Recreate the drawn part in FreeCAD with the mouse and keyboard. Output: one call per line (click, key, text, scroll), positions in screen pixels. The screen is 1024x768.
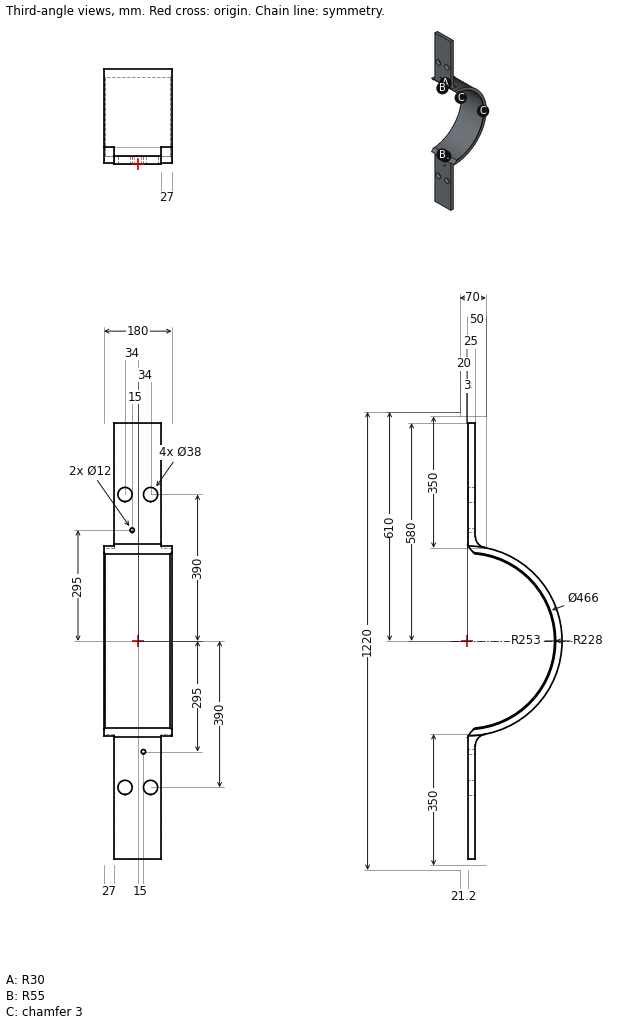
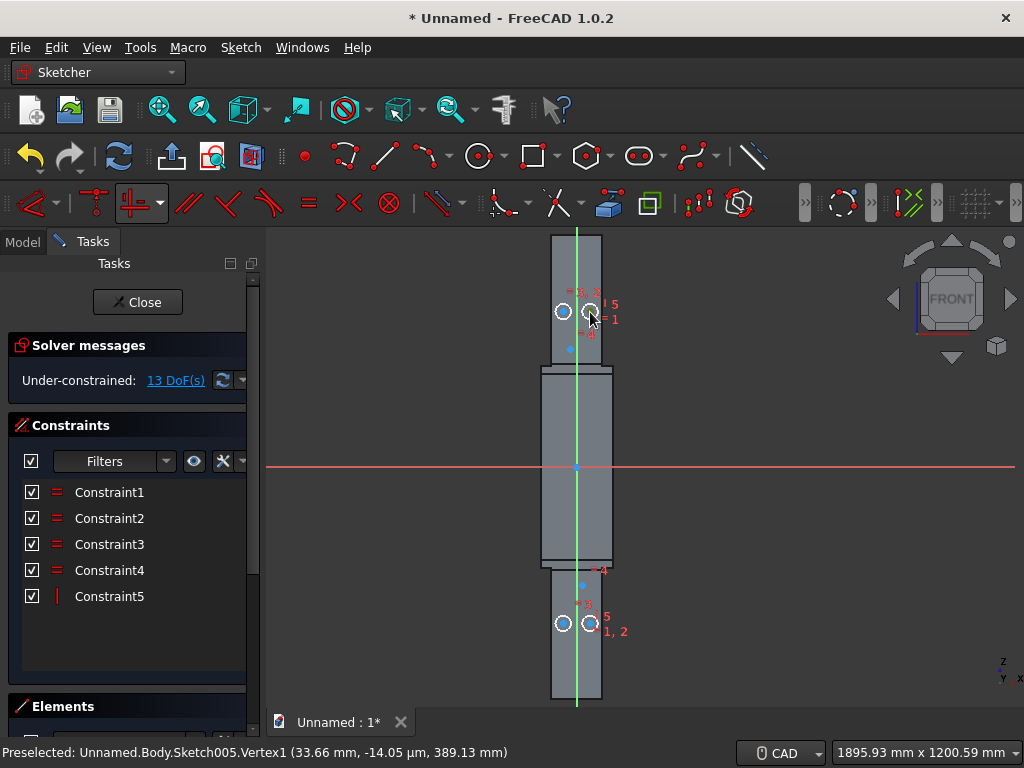
click(563, 312)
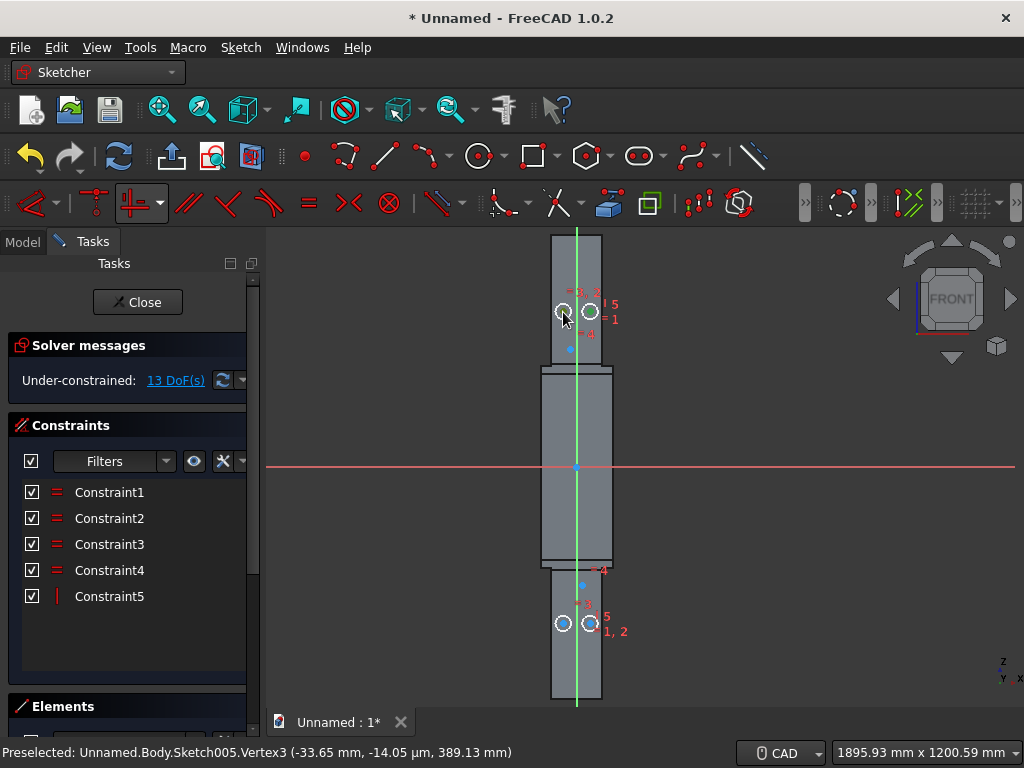
key(h)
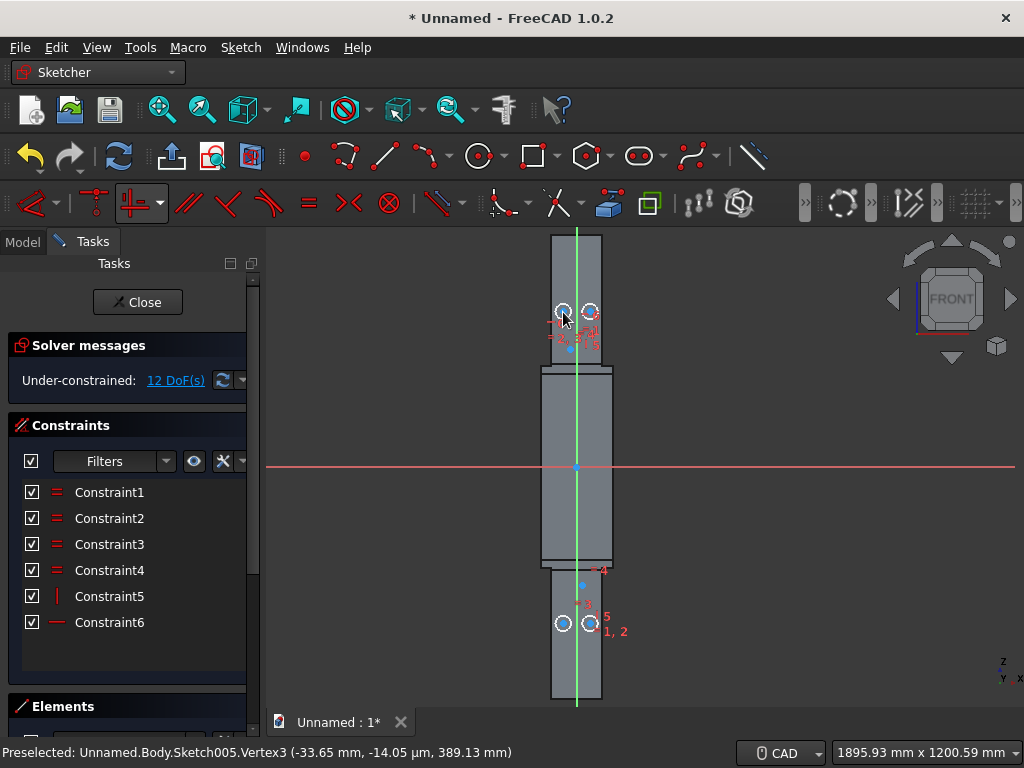
click(563, 312)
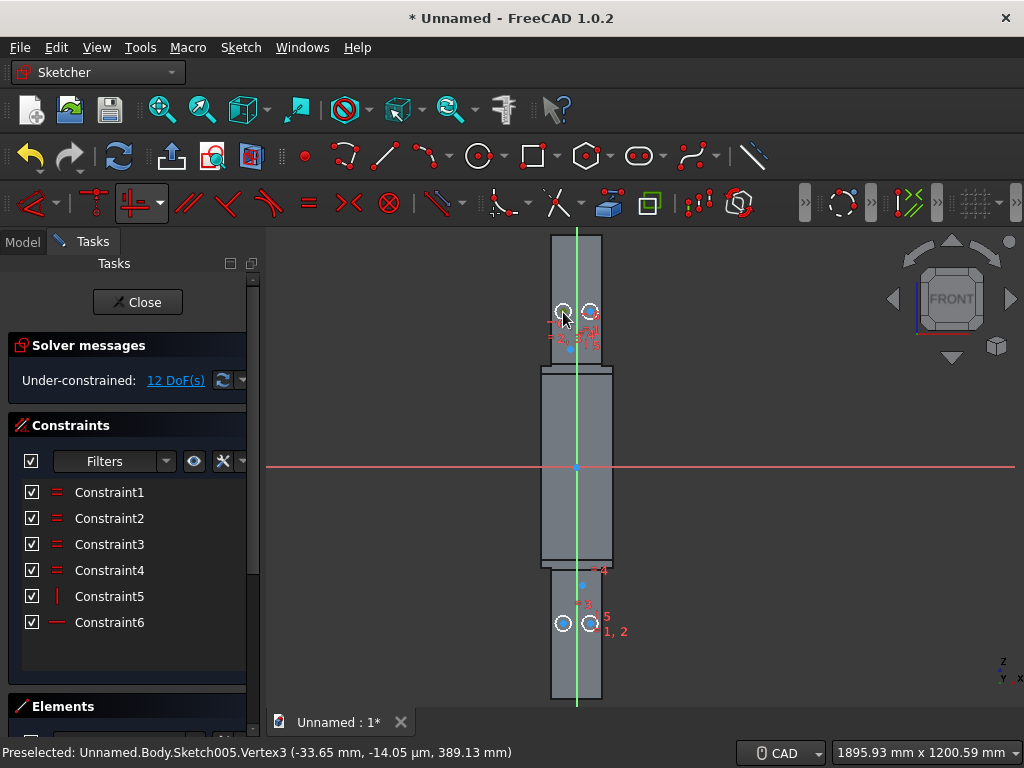
click(563, 623)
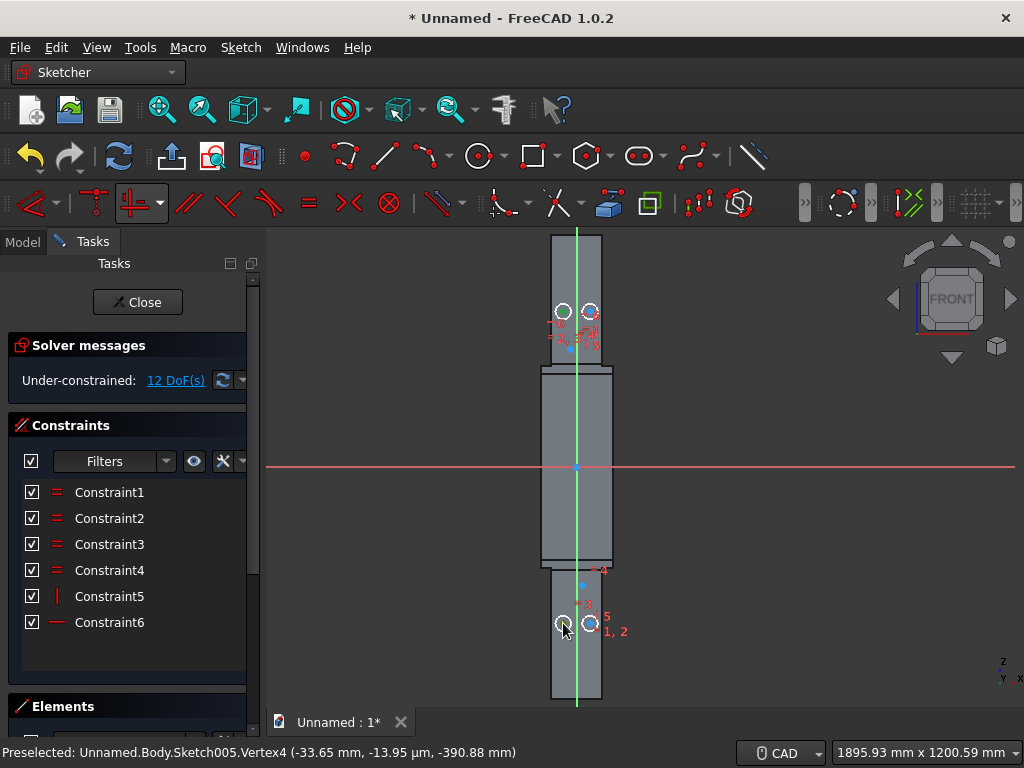
key(v)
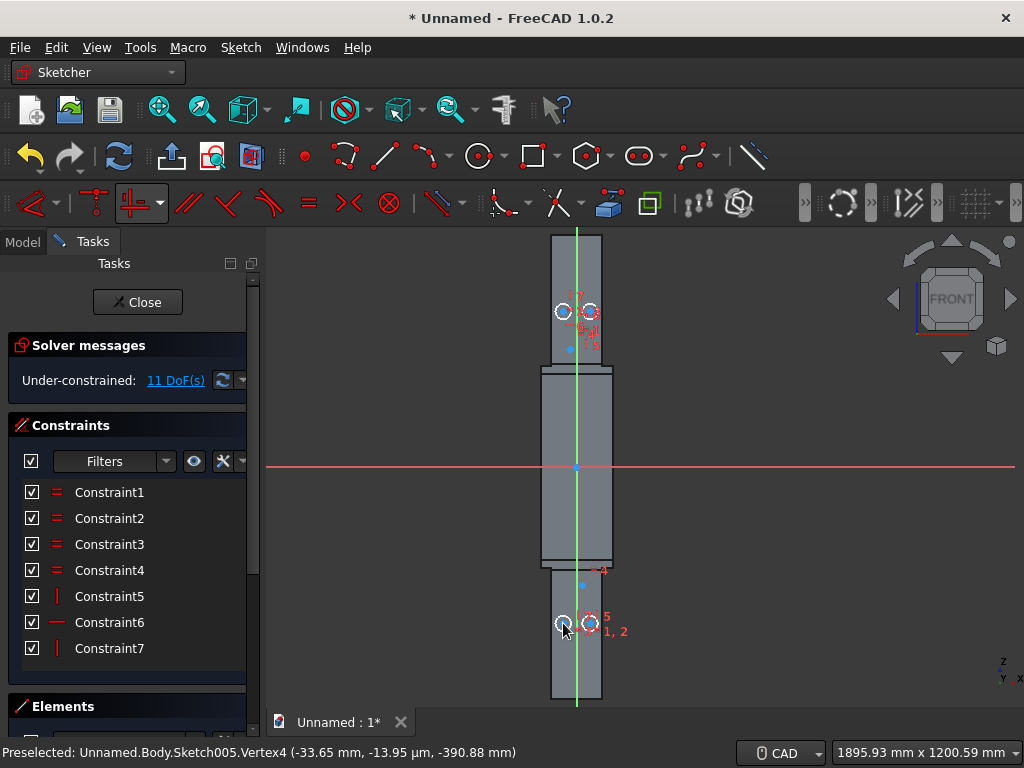
scroll(590, 623, up, 4)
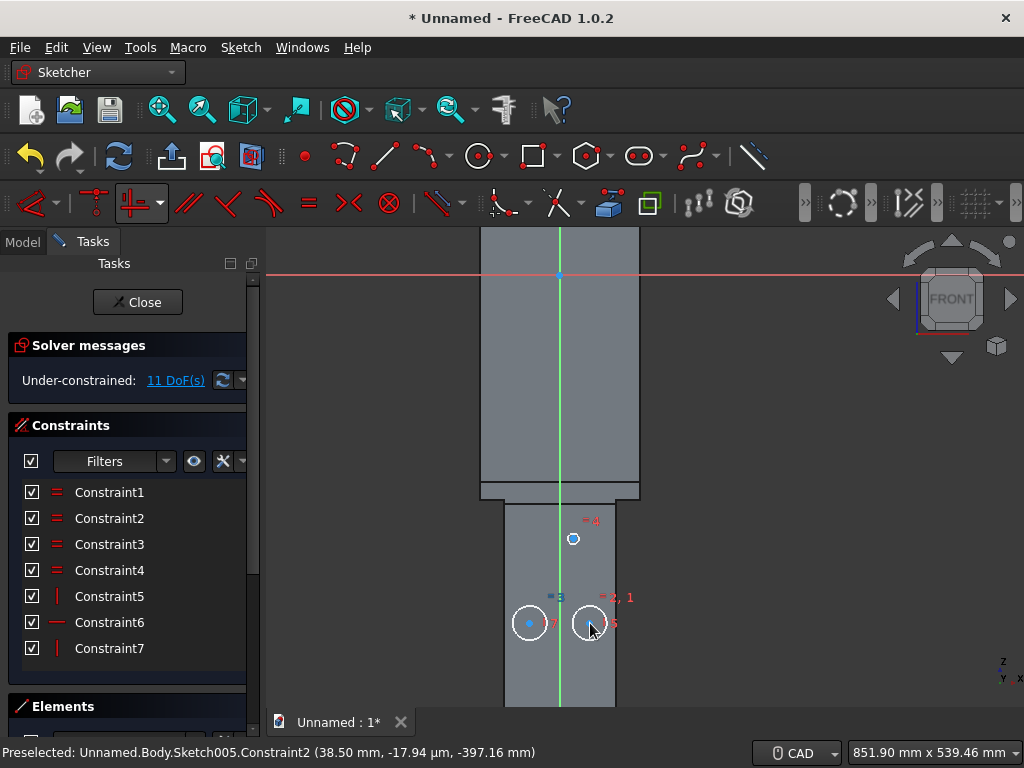
click(590, 623)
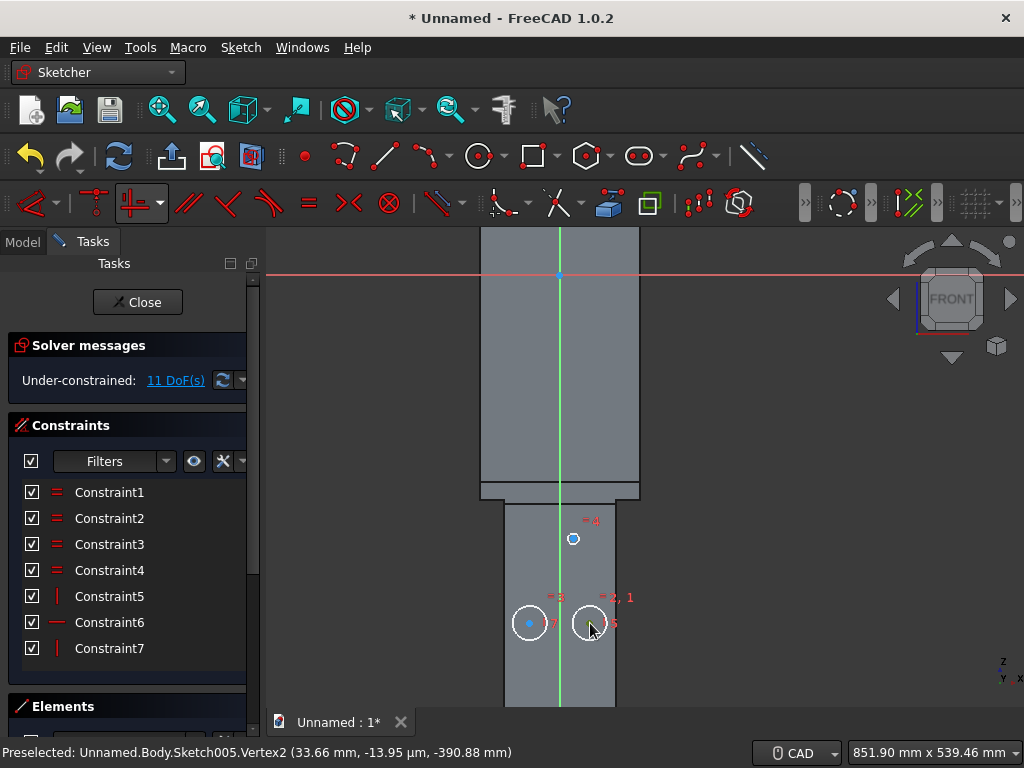
click(530, 623)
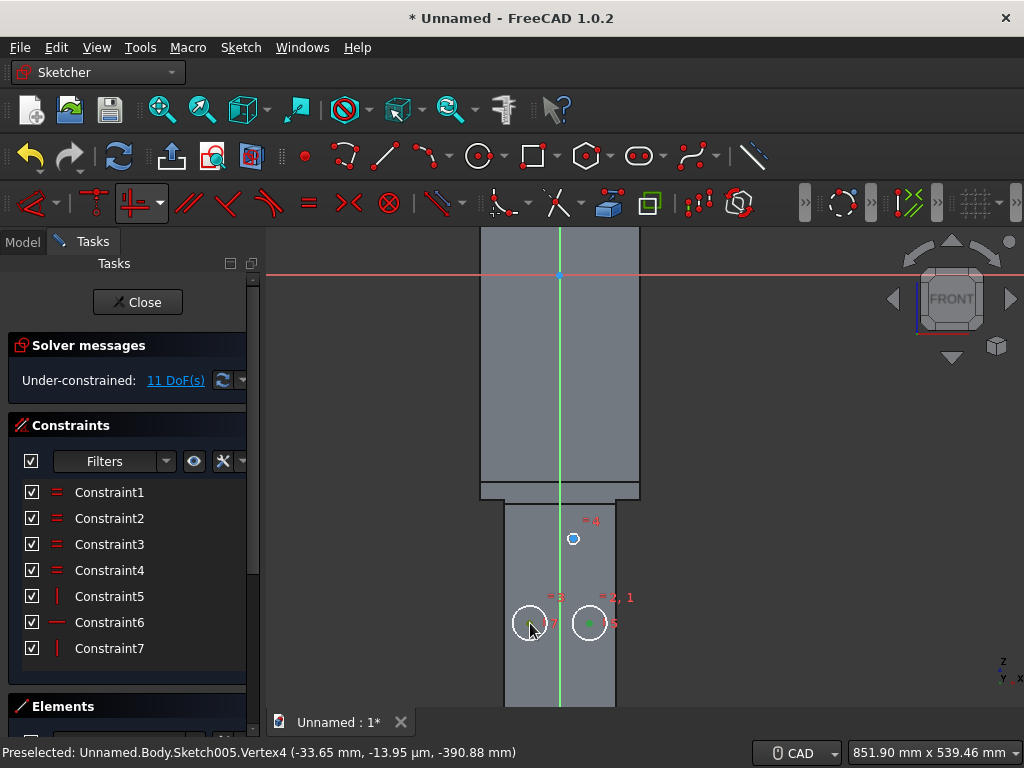
key(h)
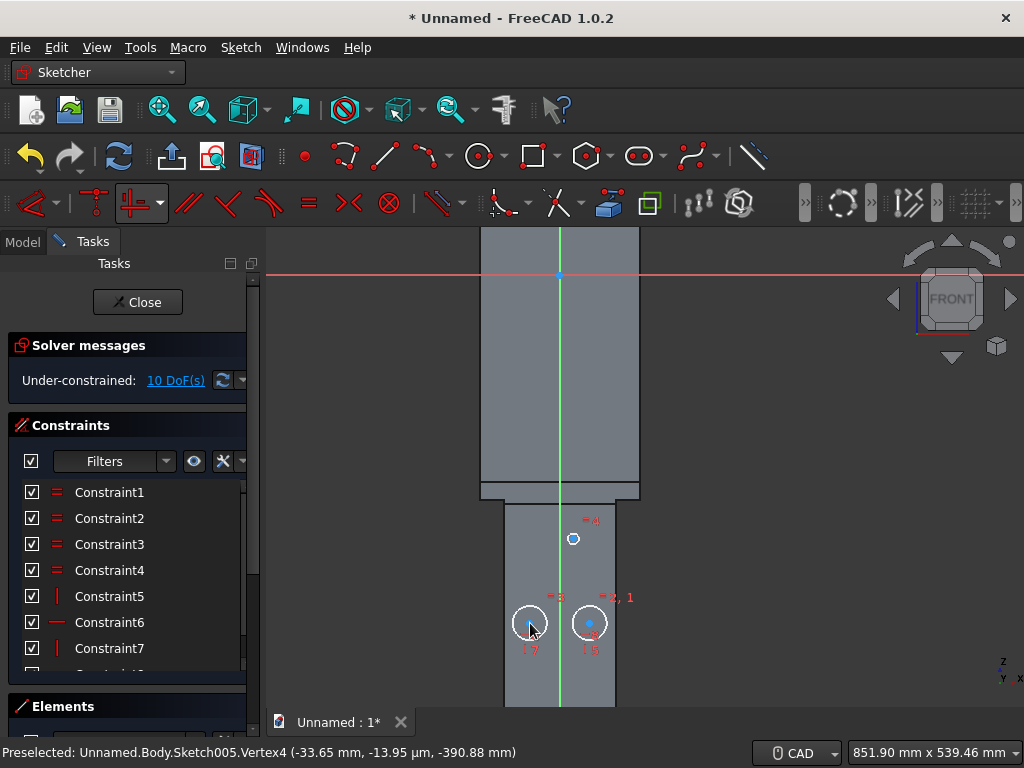
click(32, 204)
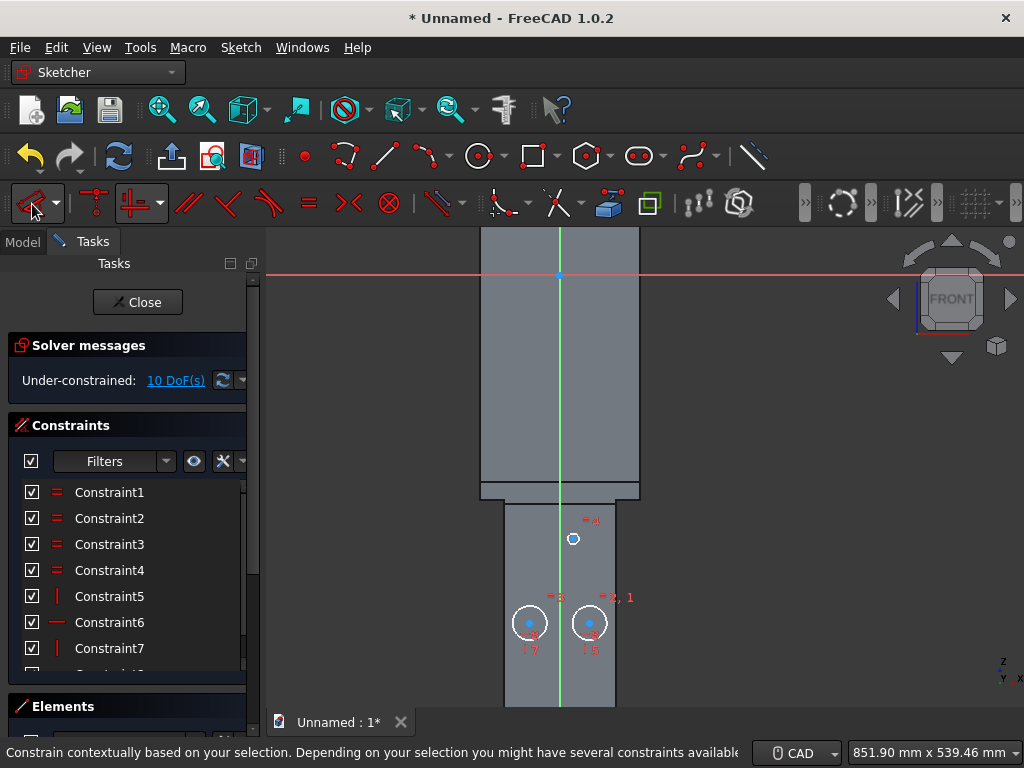
scroll(590, 623, down, 4)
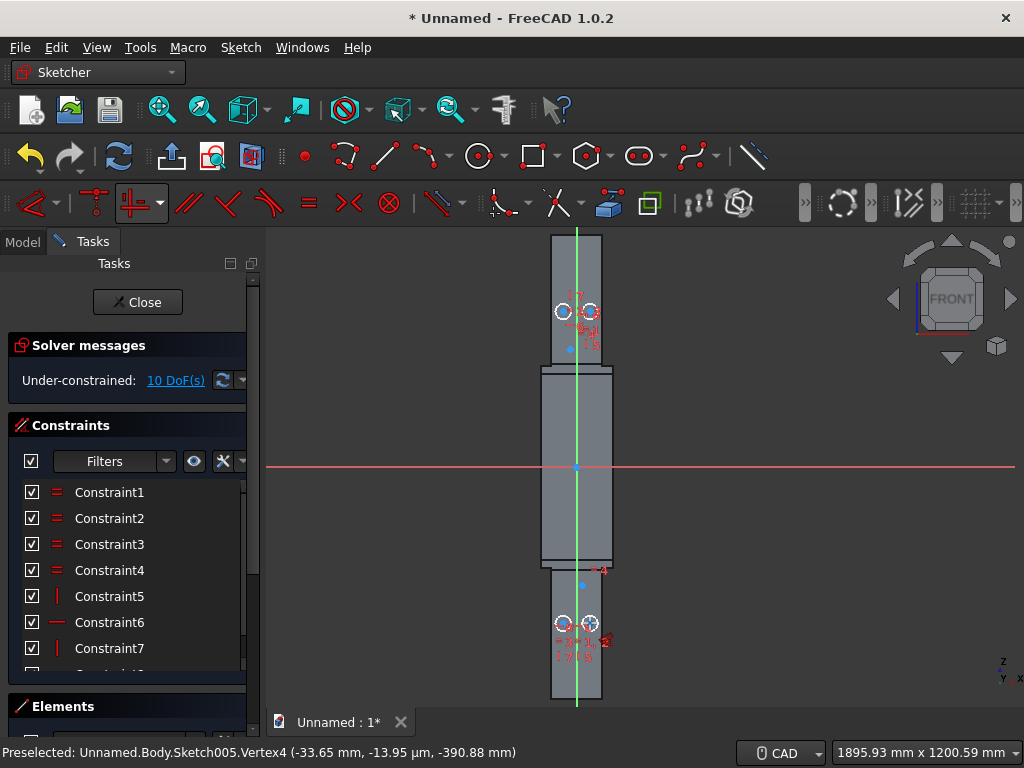
scroll(595, 306, up, 5)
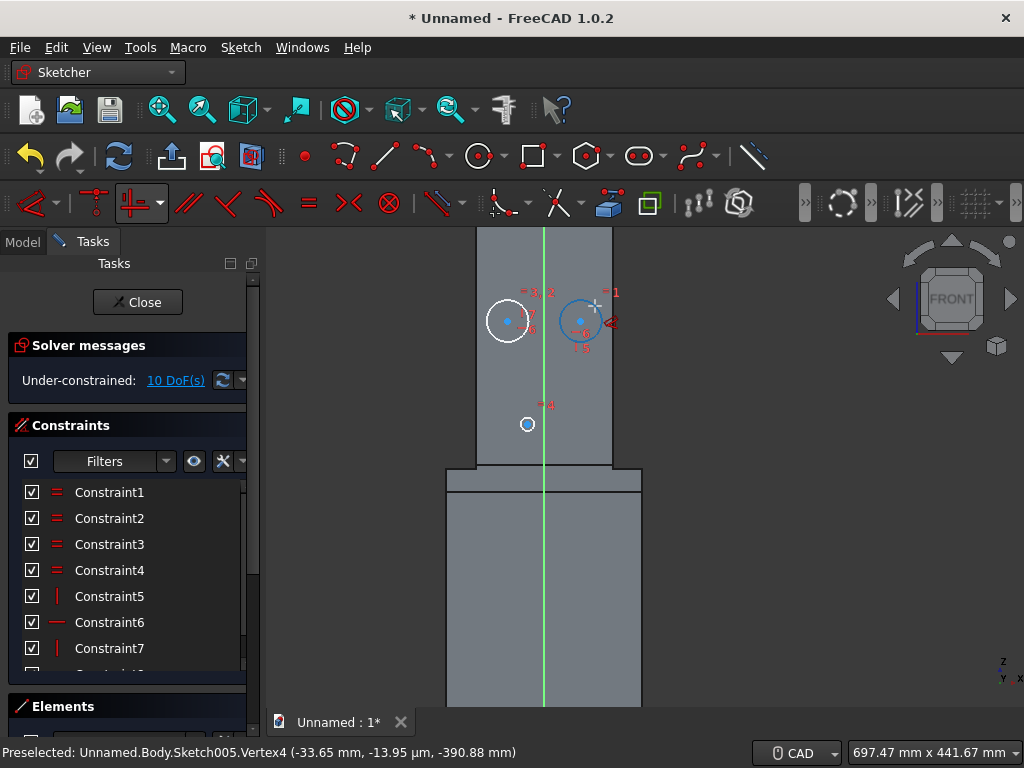
click(596, 306)
click(619, 283)